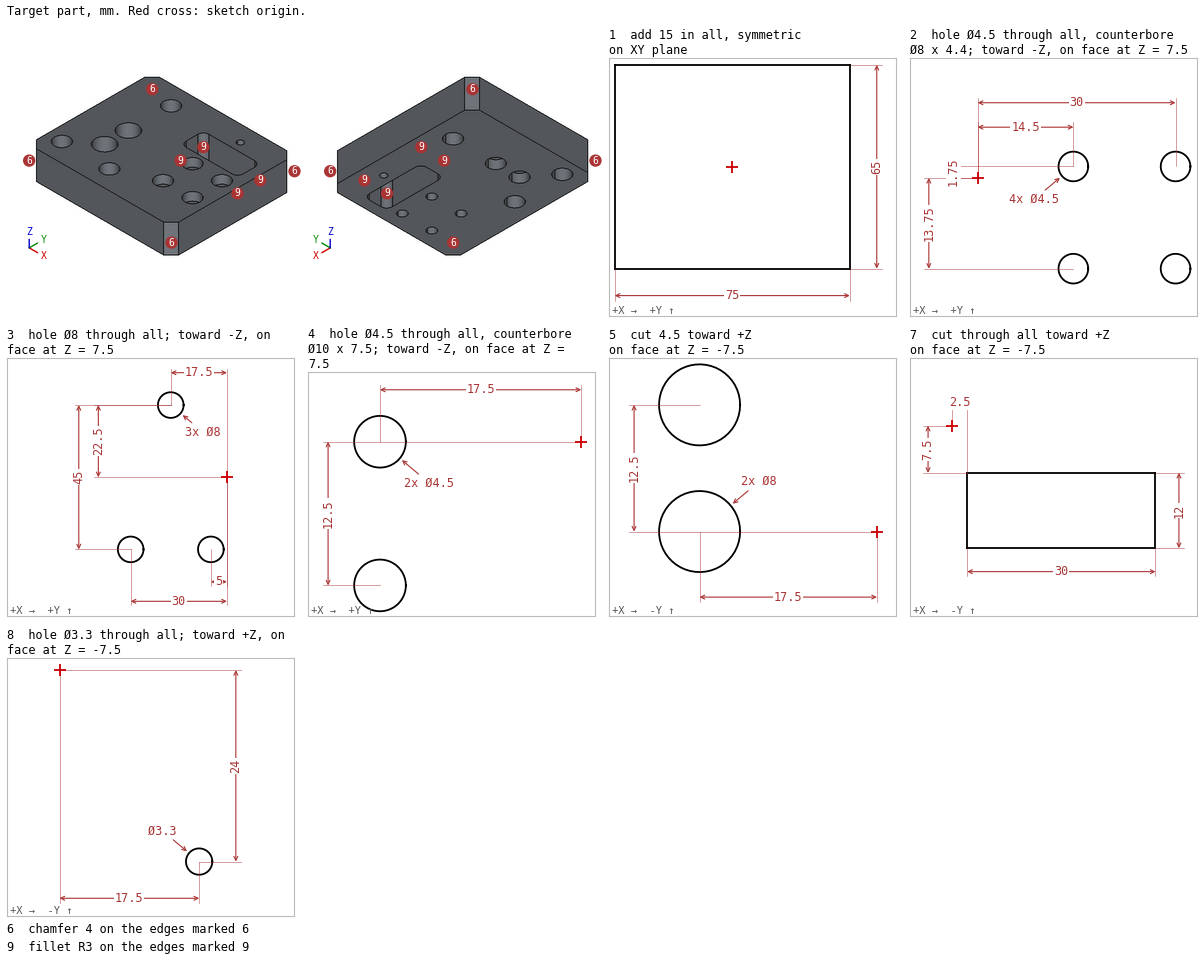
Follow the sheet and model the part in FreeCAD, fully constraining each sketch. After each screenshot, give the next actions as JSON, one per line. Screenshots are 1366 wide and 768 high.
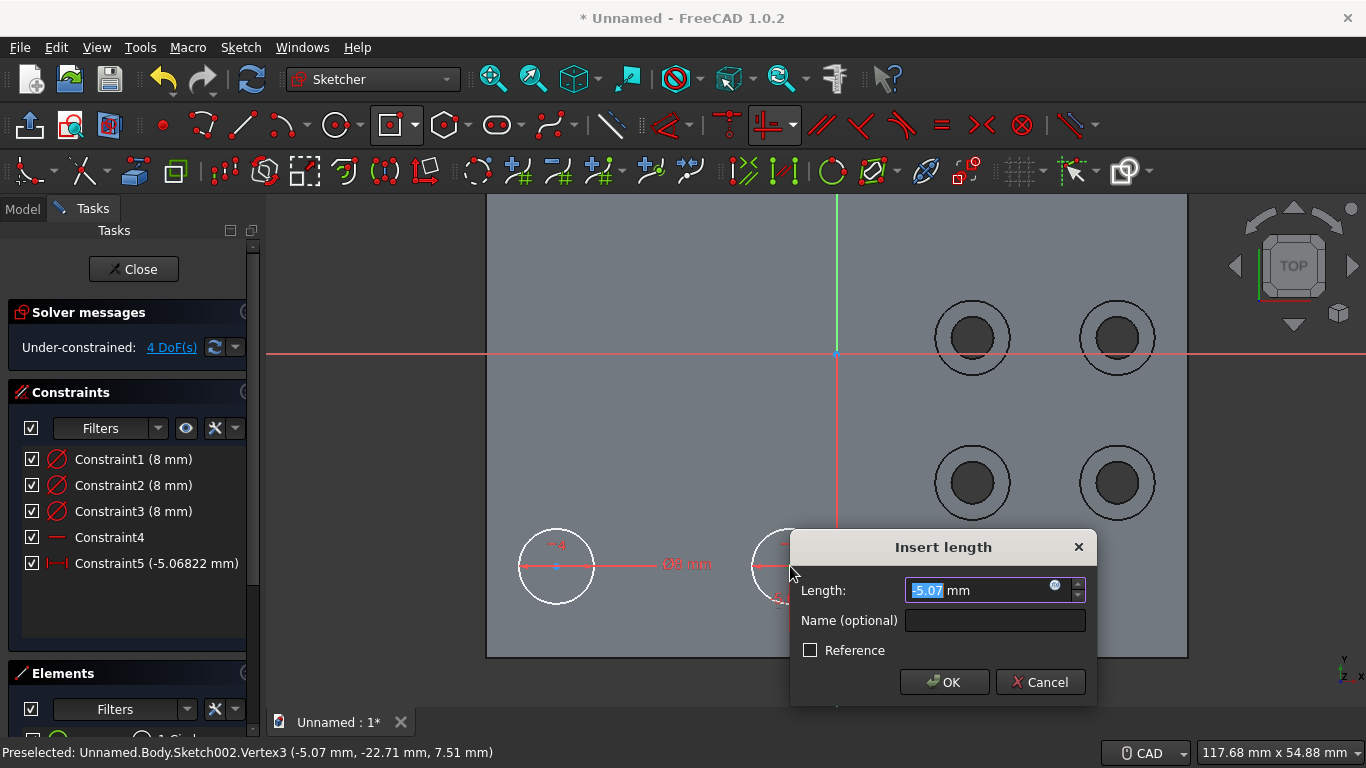
{"action": "type", "text": "-5"}
{"action": "key", "text": "Return"}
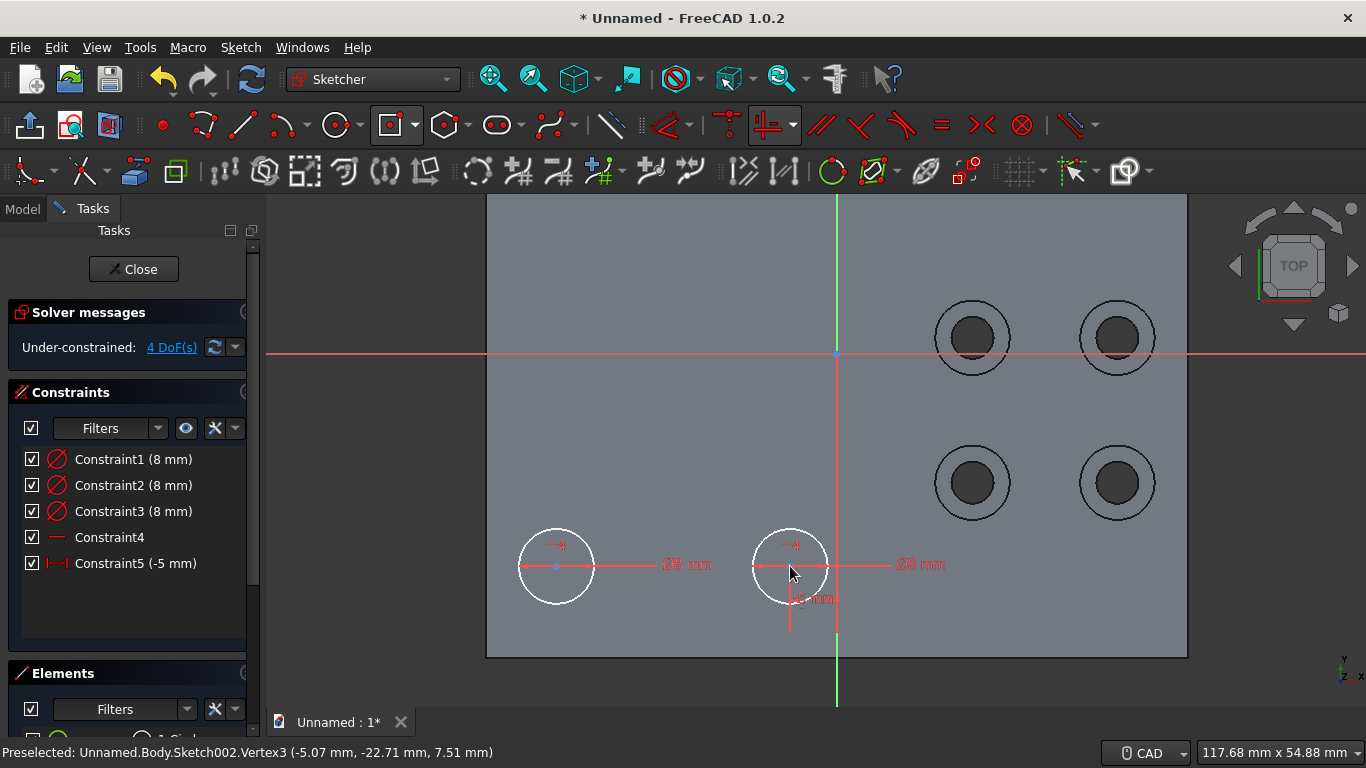
{"action": "left_click", "coordinate": [556, 566]}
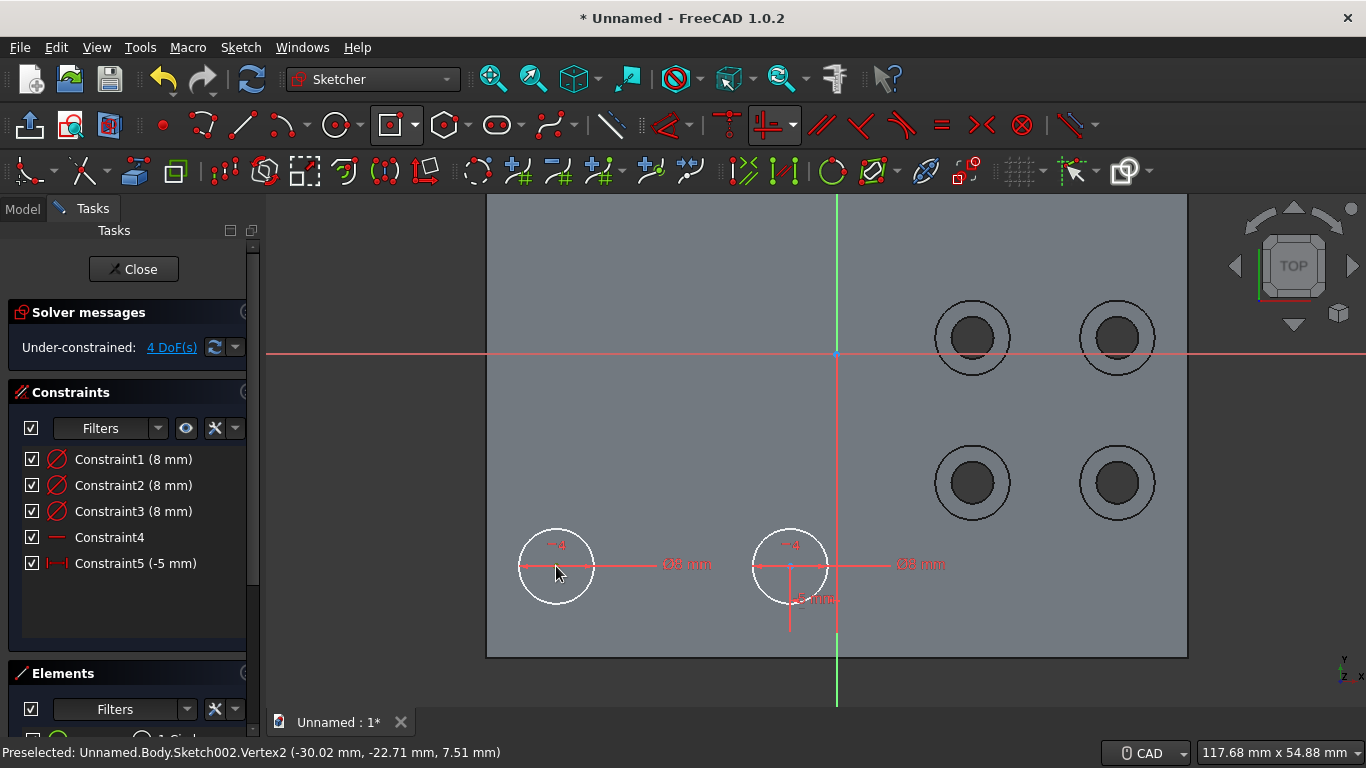
{"action": "key", "text": "l"}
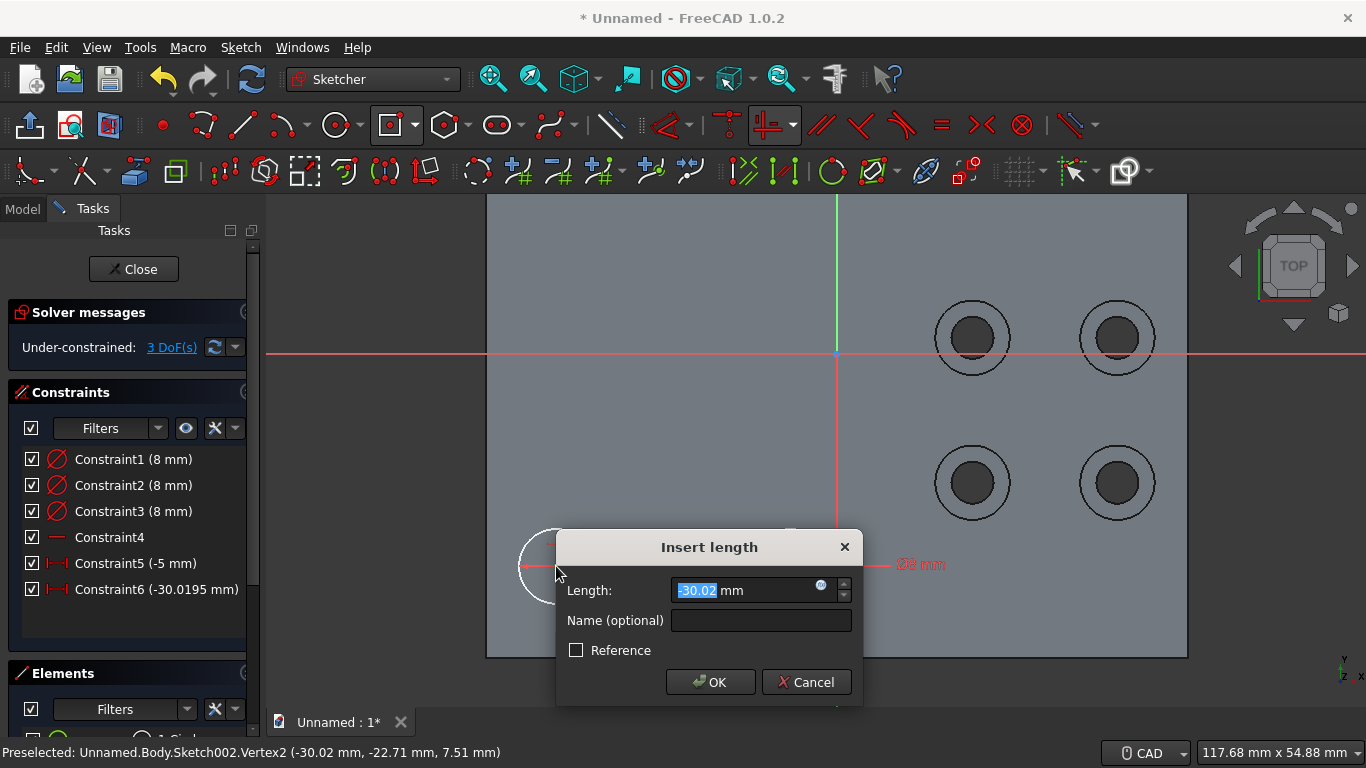
{"action": "type", "text": "-30"}
{"action": "key", "text": "Return"}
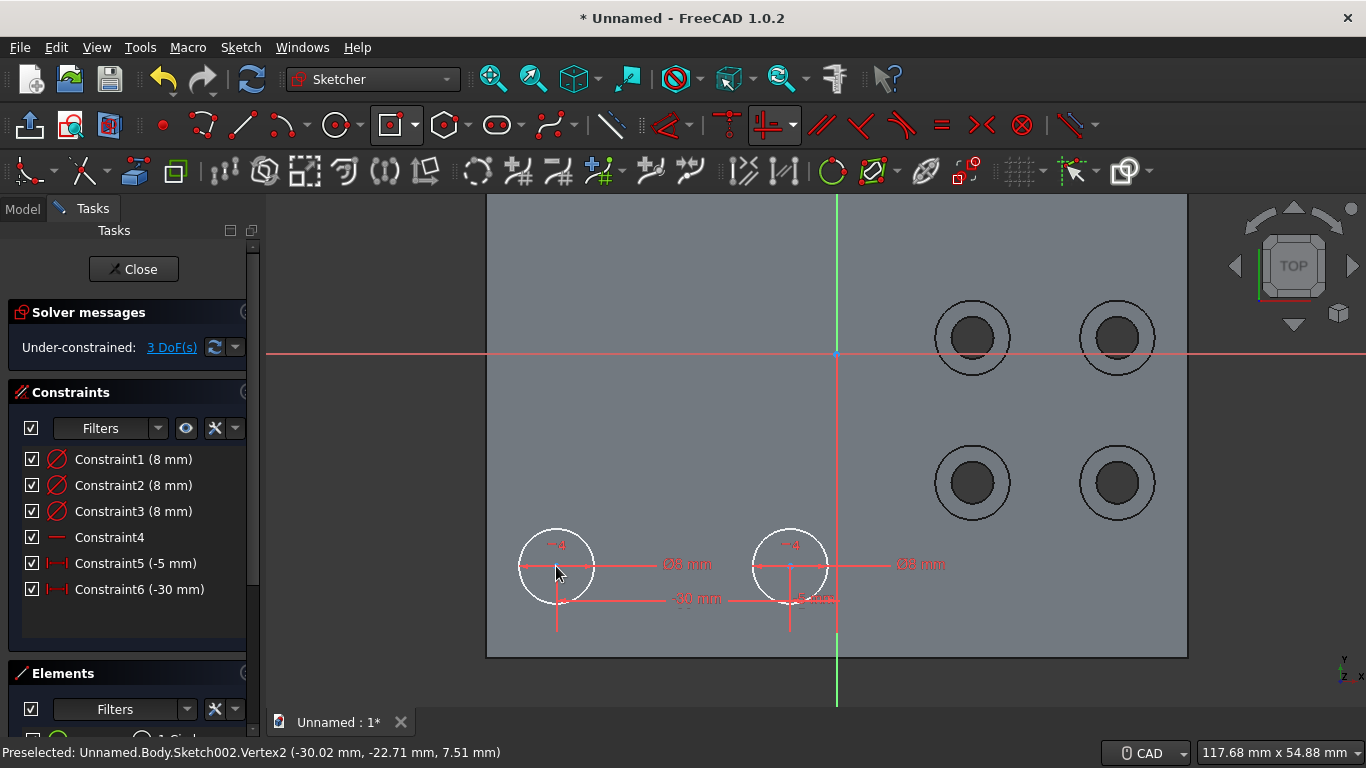
{"action": "scroll", "coordinate": [889, 646], "scroll_direction": "down", "scroll_amount": 2}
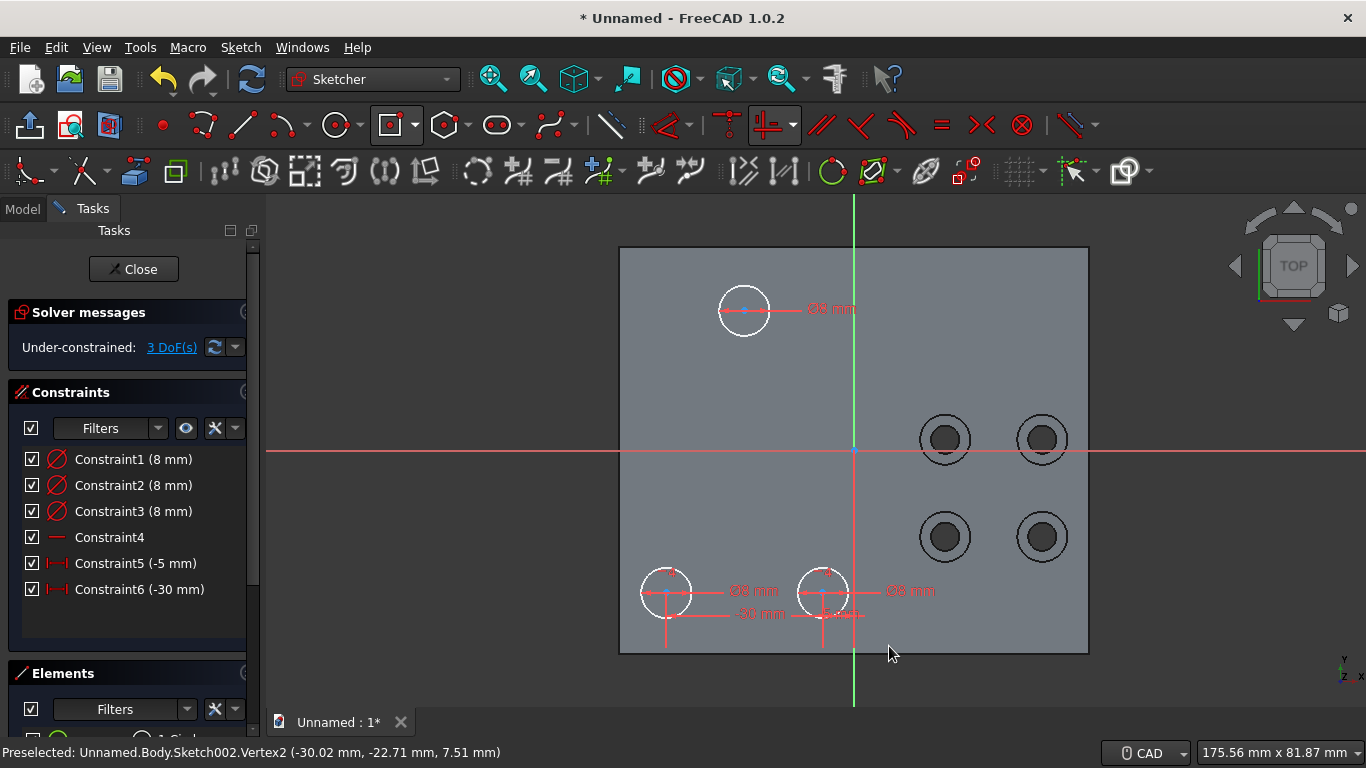
{"action": "left_click", "coordinate": [744, 311]}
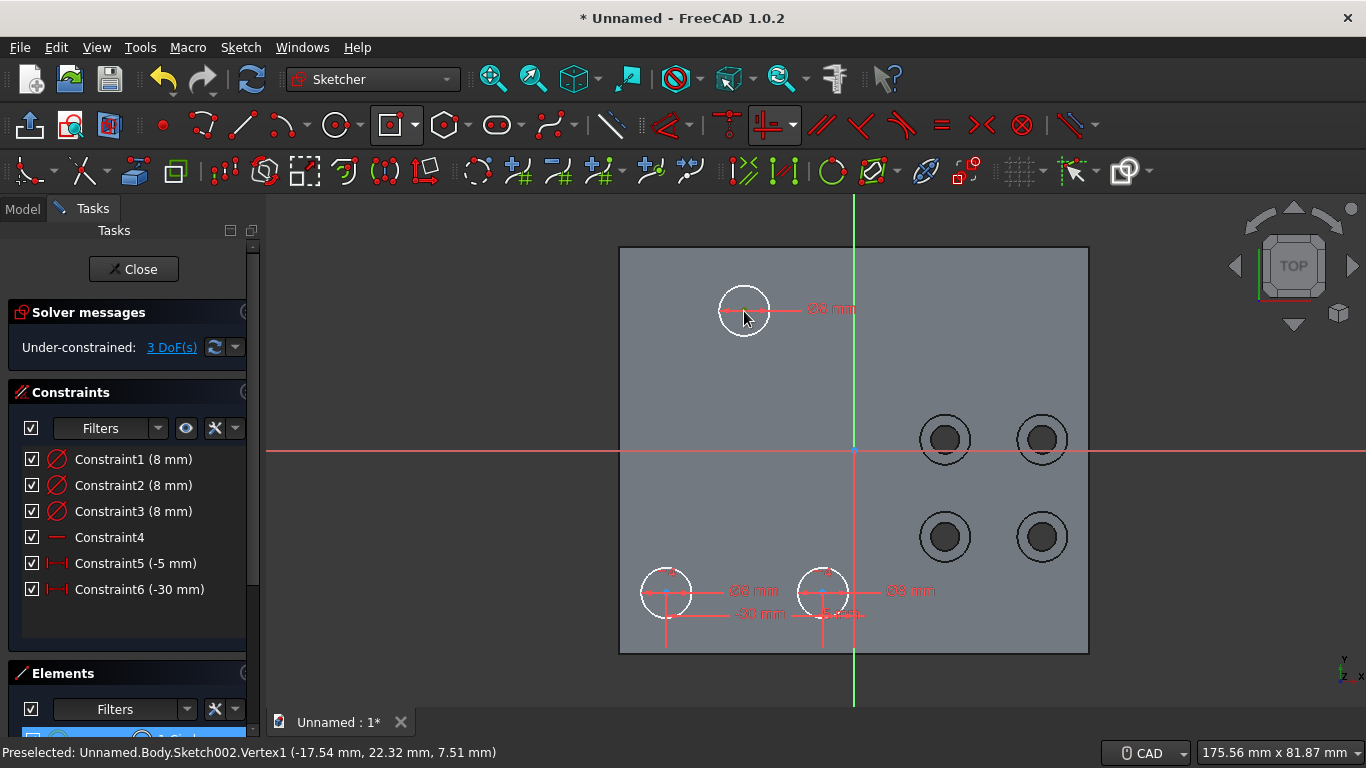
{"action": "left_click", "coordinate": [666, 593]}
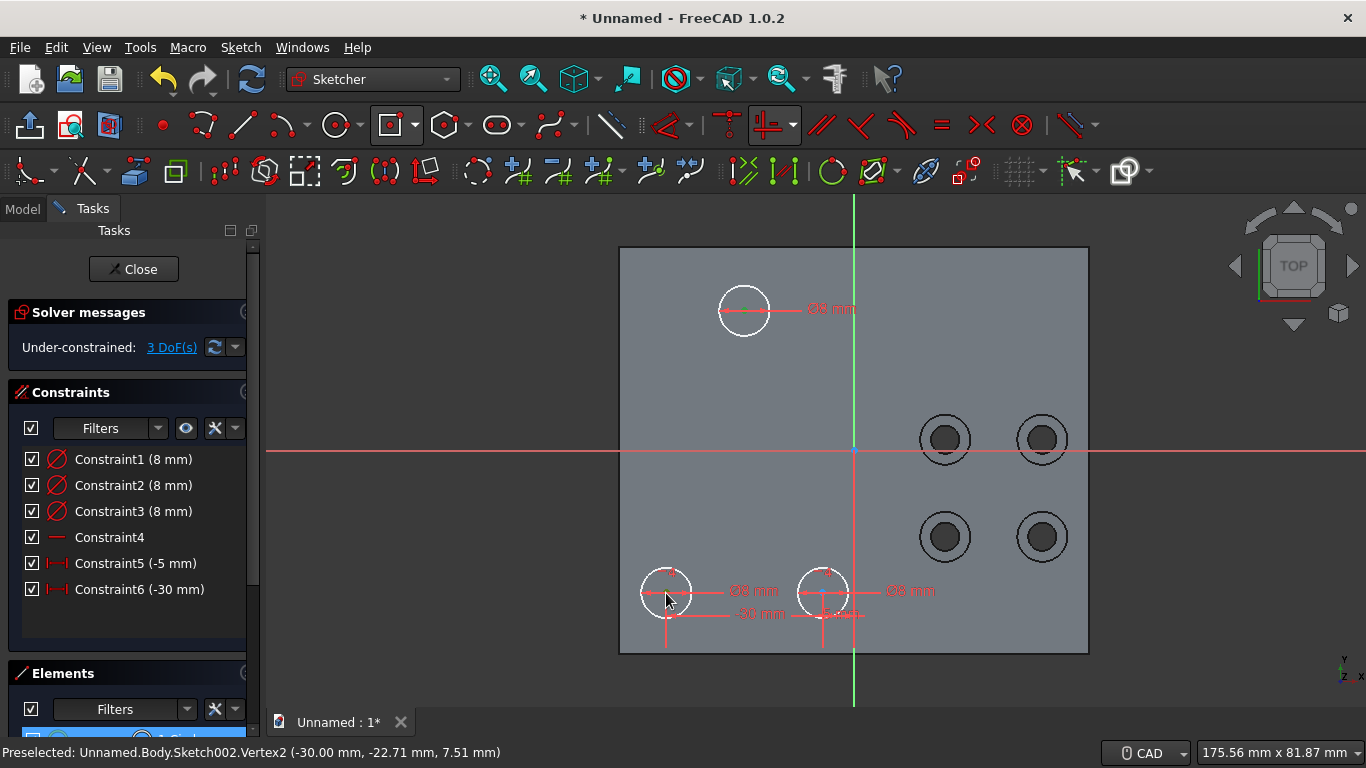
{"action": "key", "text": "i"}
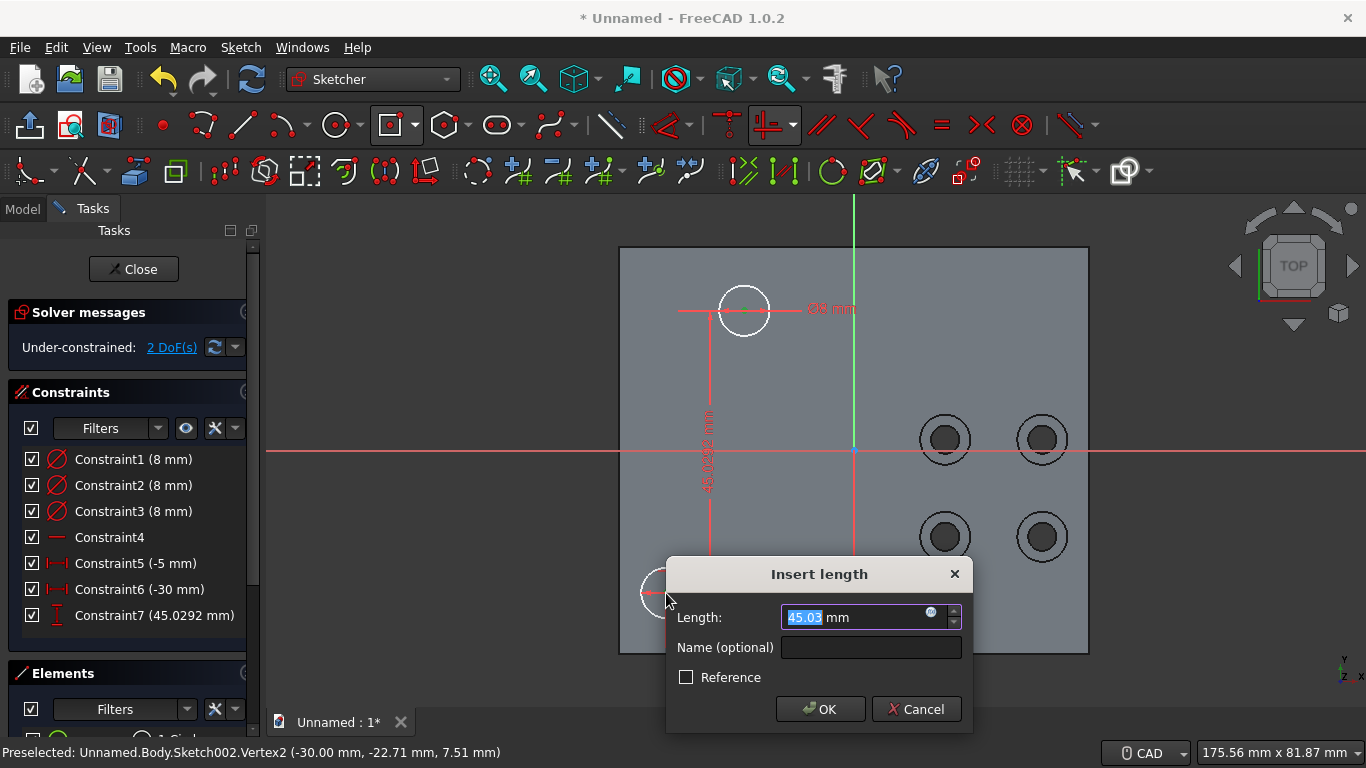
{"action": "type", "text": "45"}
{"action": "key", "text": "Return"}